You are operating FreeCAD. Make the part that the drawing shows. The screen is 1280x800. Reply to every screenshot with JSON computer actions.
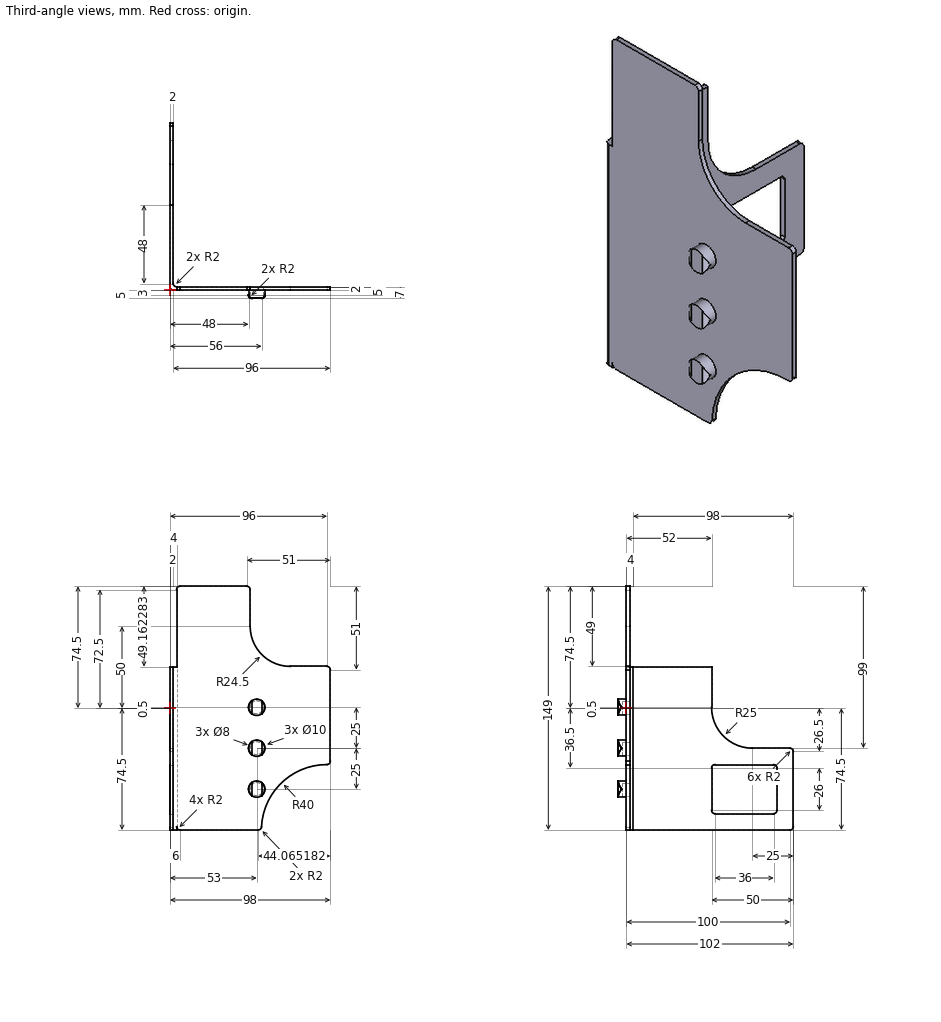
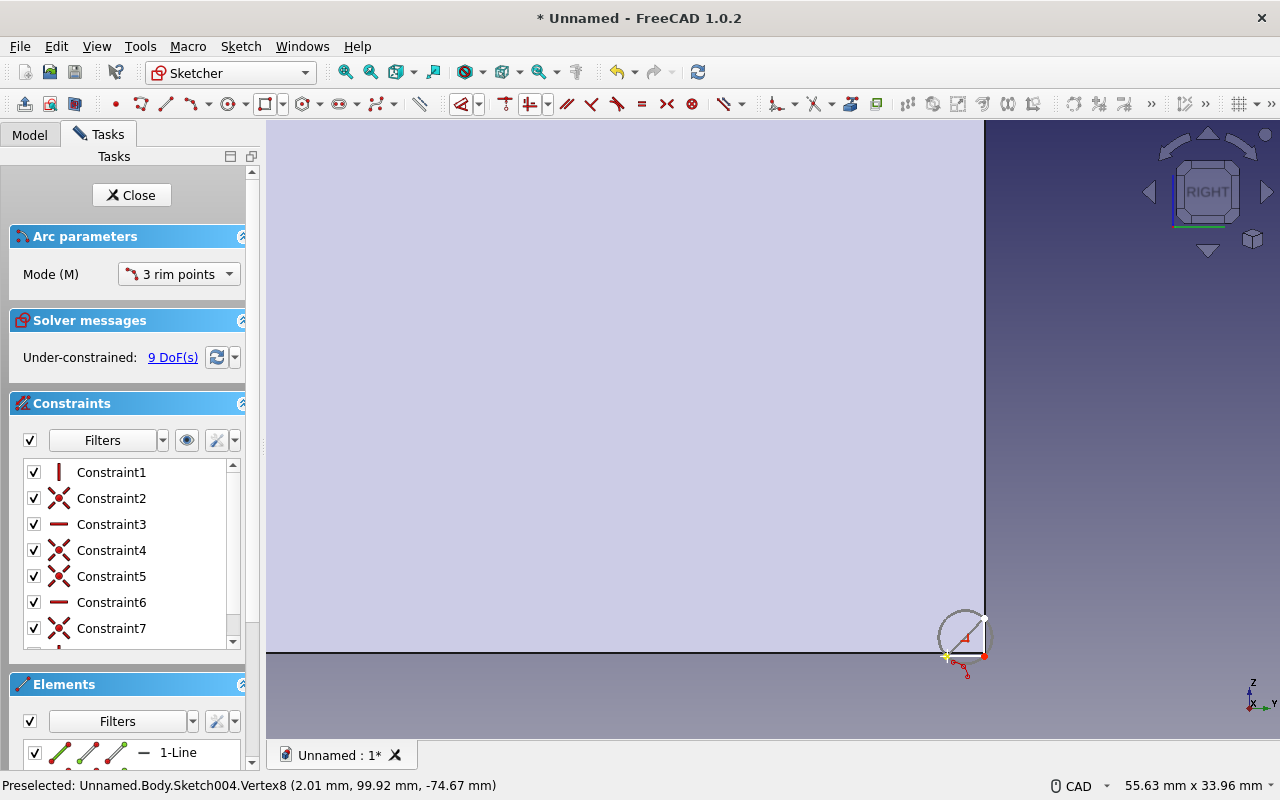
{"action": "scroll", "coordinate": [974, 642], "scroll_direction": "up", "scroll_amount": 2}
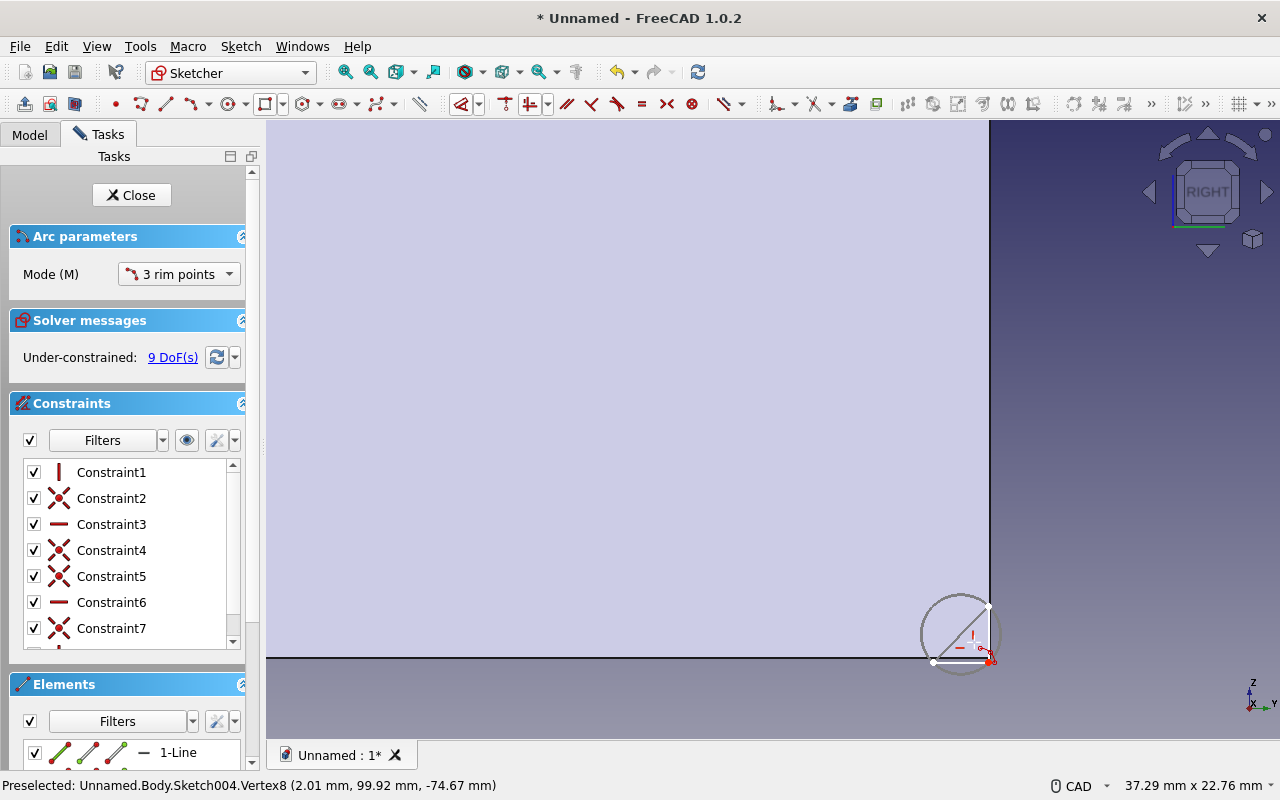
{"action": "left_click", "coordinate": [974, 642]}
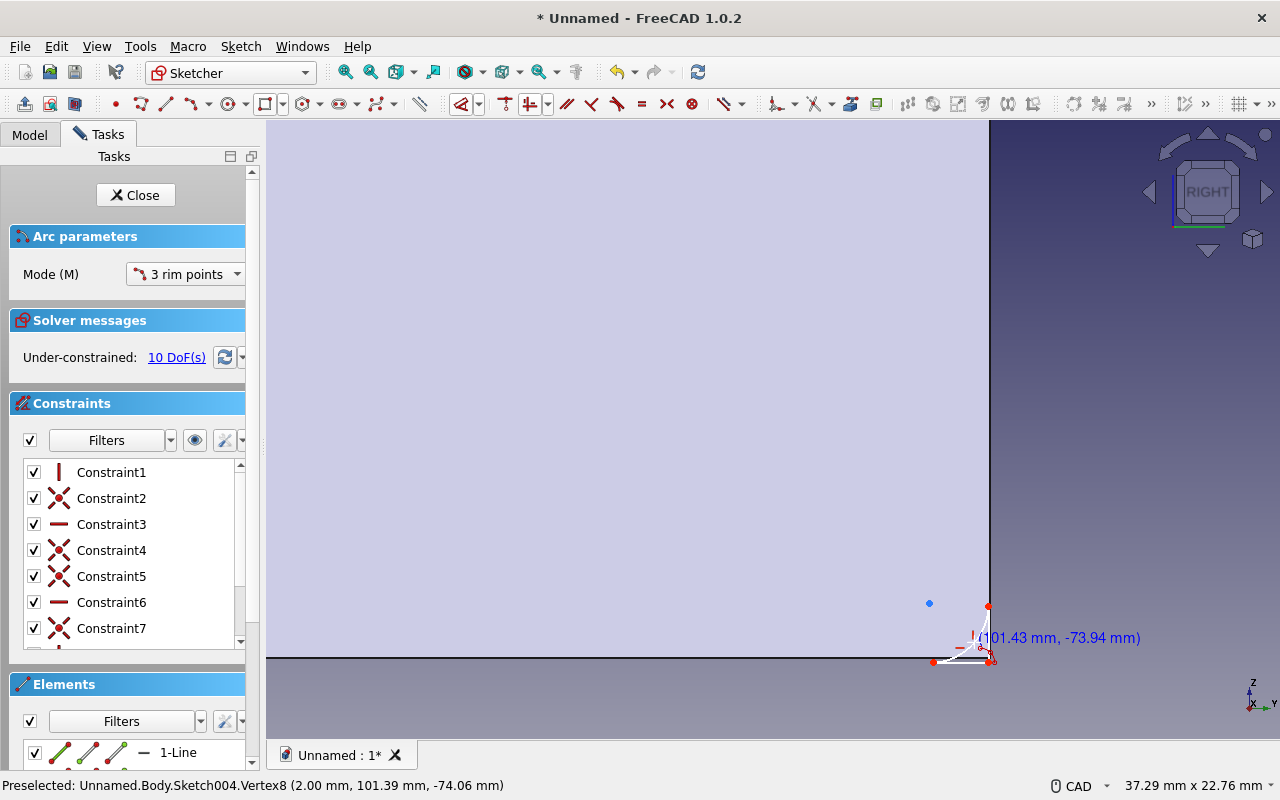
{"action": "key", "text": "g l"}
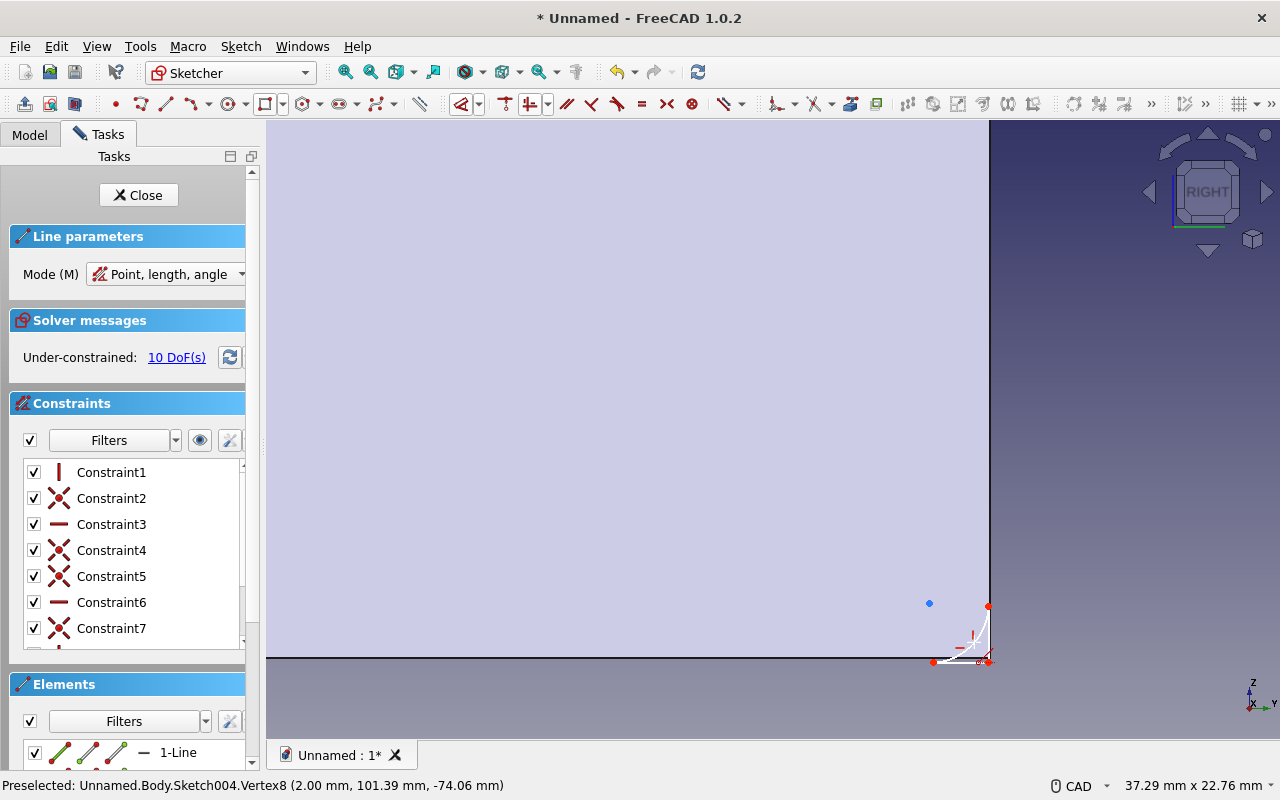
{"action": "scroll", "coordinate": [983, 628], "scroll_direction": "down", "scroll_amount": 8}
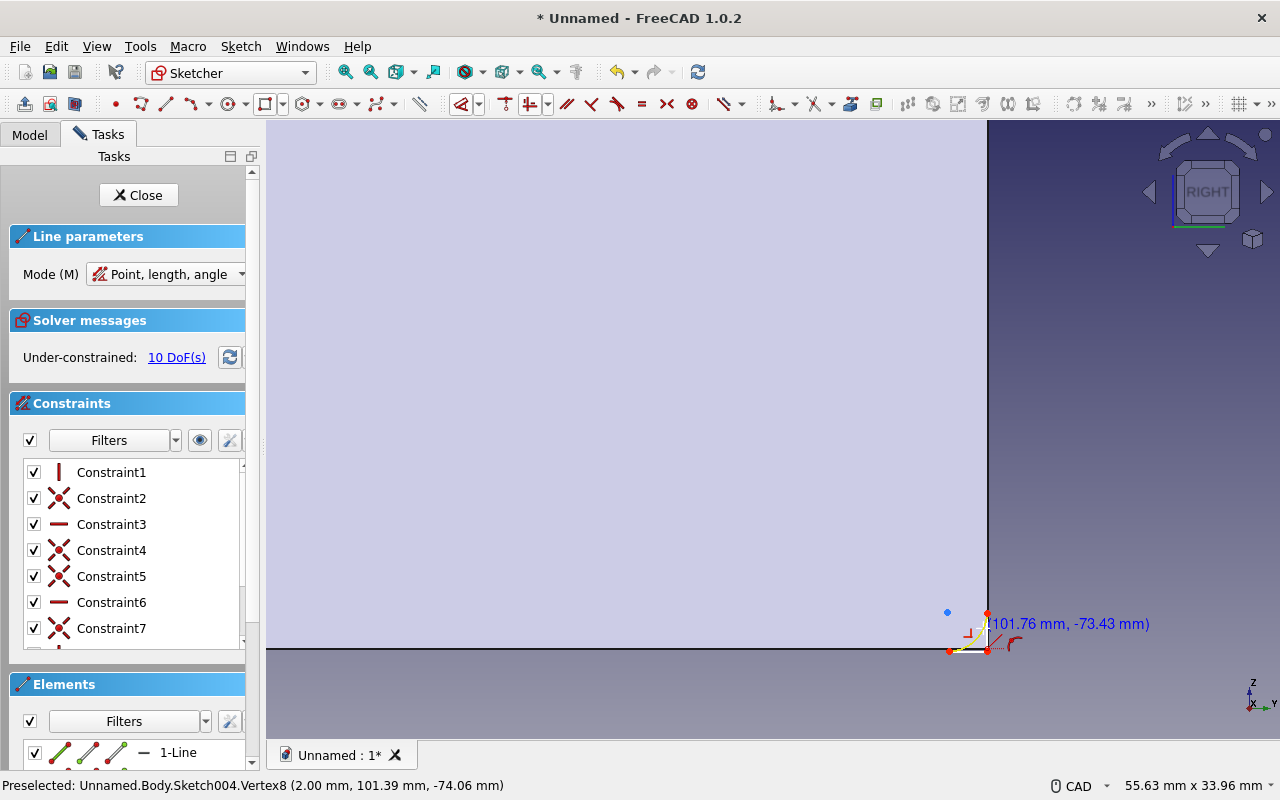
{"action": "left_click", "coordinate": [710, 426]}
{"action": "left_click", "coordinate": [710, 569]}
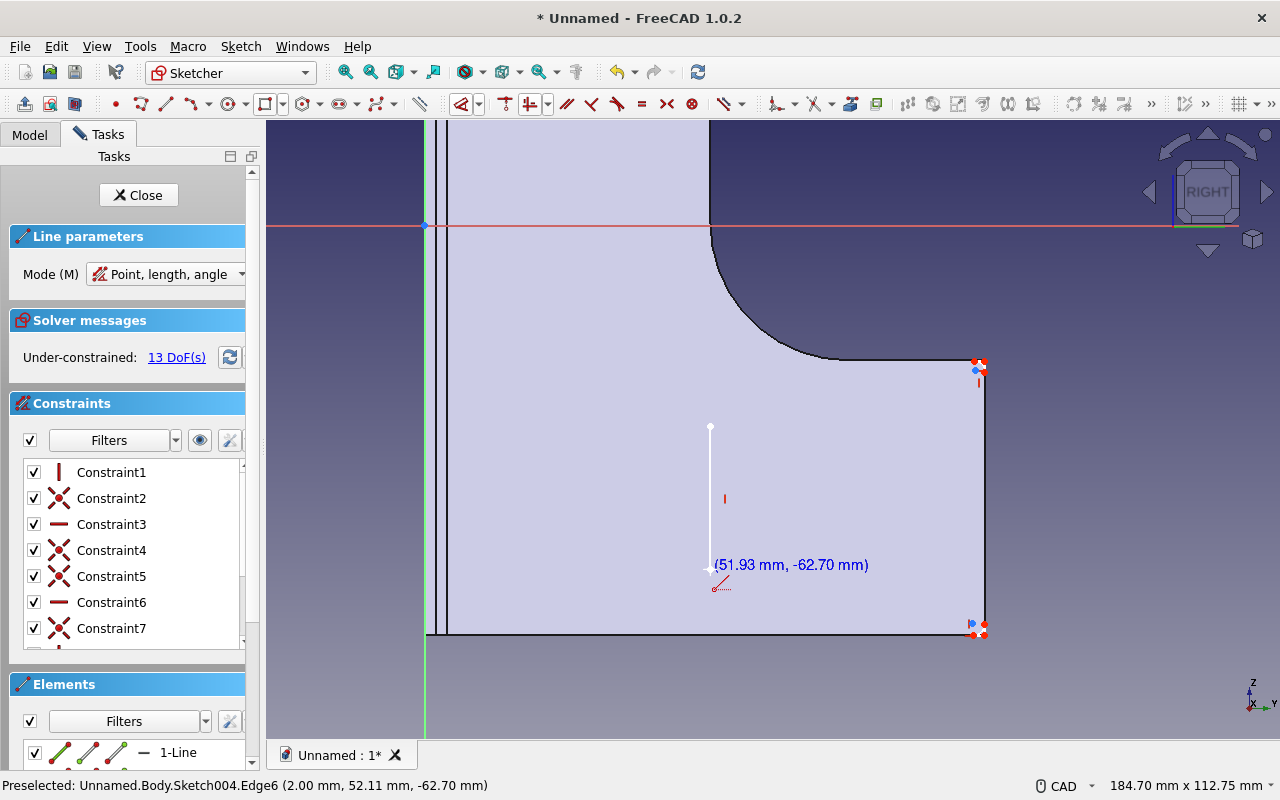
{"action": "left_click", "coordinate": [721, 580]}
{"action": "left_click", "coordinate": [919, 580]}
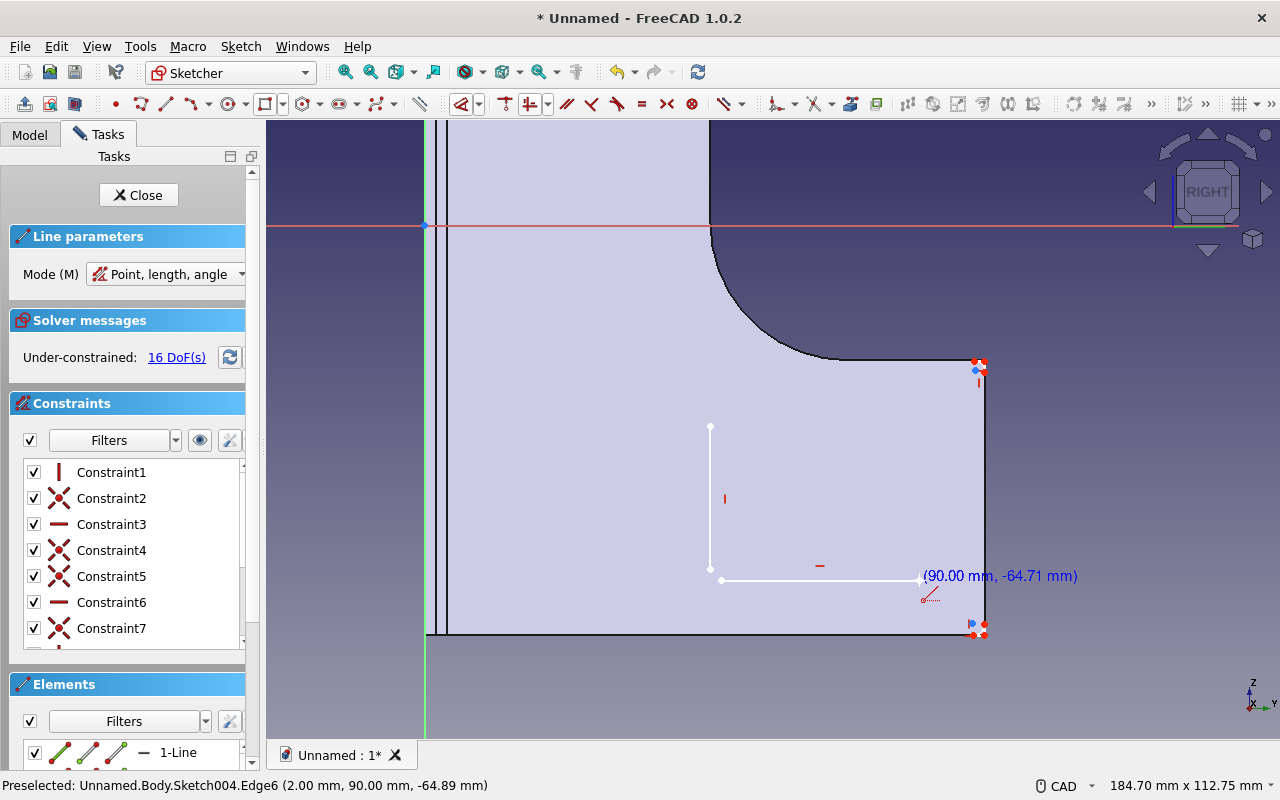
{"action": "left_click", "coordinate": [930, 569]}
{"action": "left_click", "coordinate": [930, 426]}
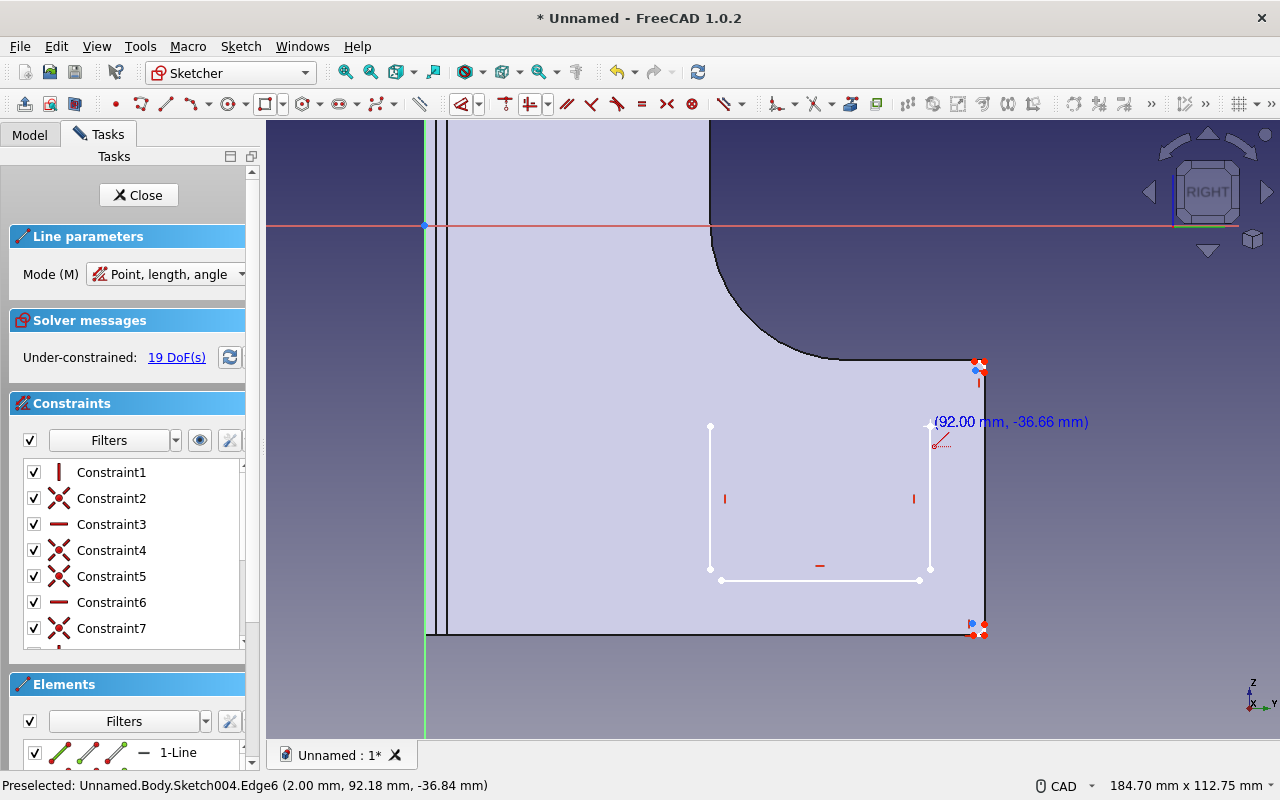
{"action": "left_click", "coordinate": [919, 415]}
{"action": "left_click", "coordinate": [721, 415]}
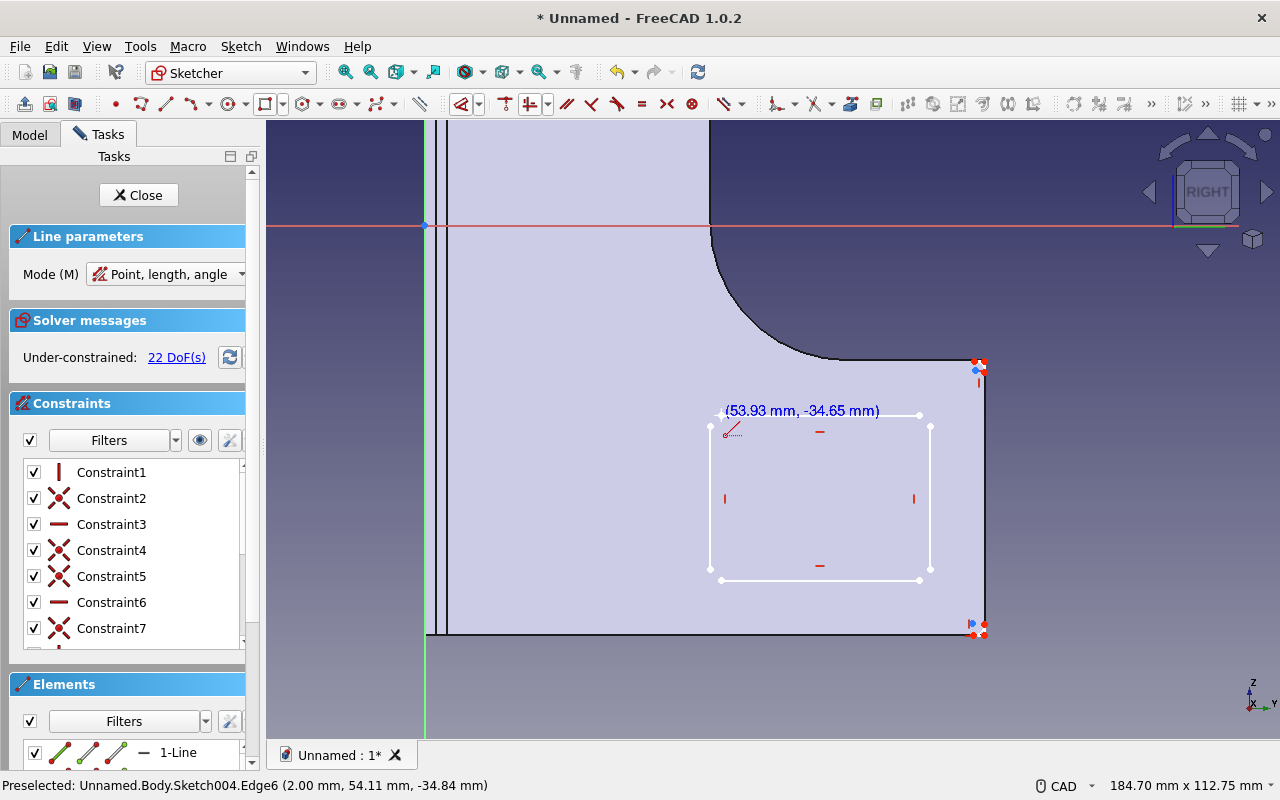
{"action": "key", "text": "g 3 a"}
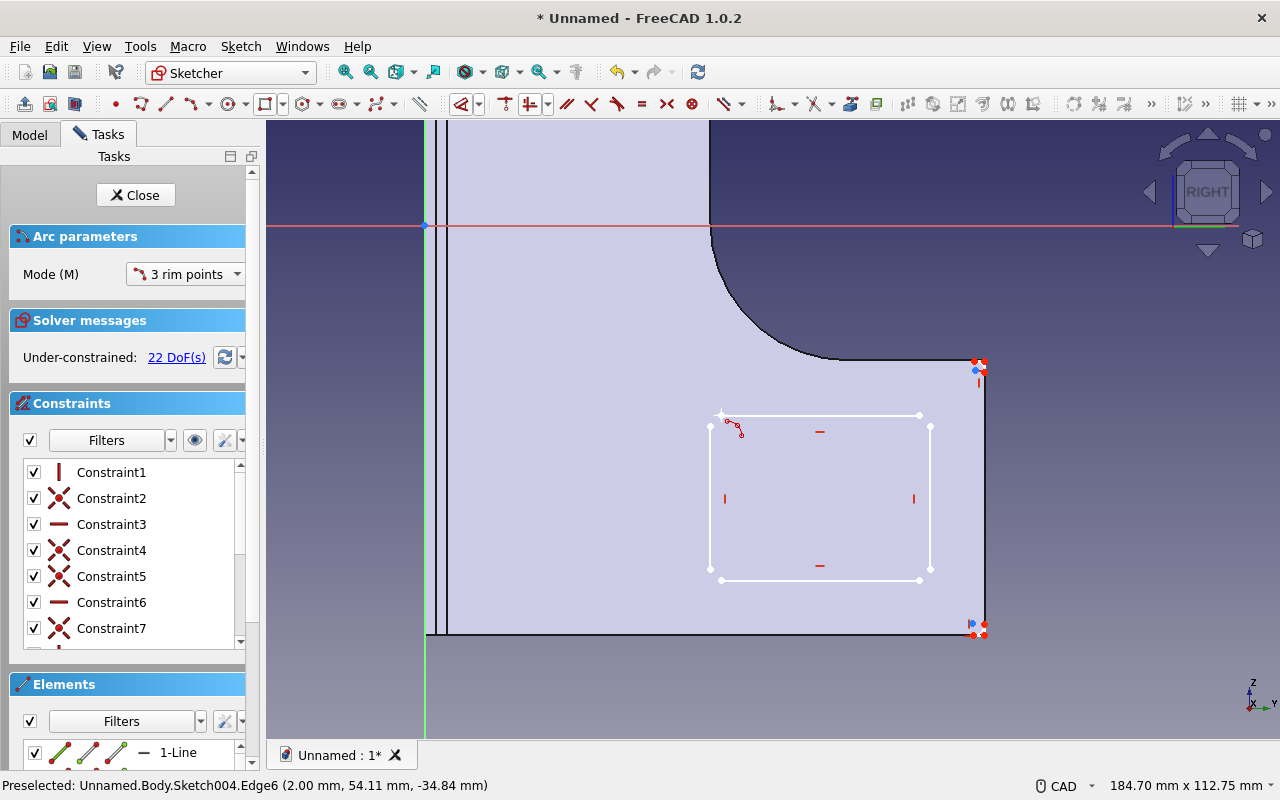
{"action": "left_click", "coordinate": [710, 570]}
{"action": "left_click", "coordinate": [721, 581]}